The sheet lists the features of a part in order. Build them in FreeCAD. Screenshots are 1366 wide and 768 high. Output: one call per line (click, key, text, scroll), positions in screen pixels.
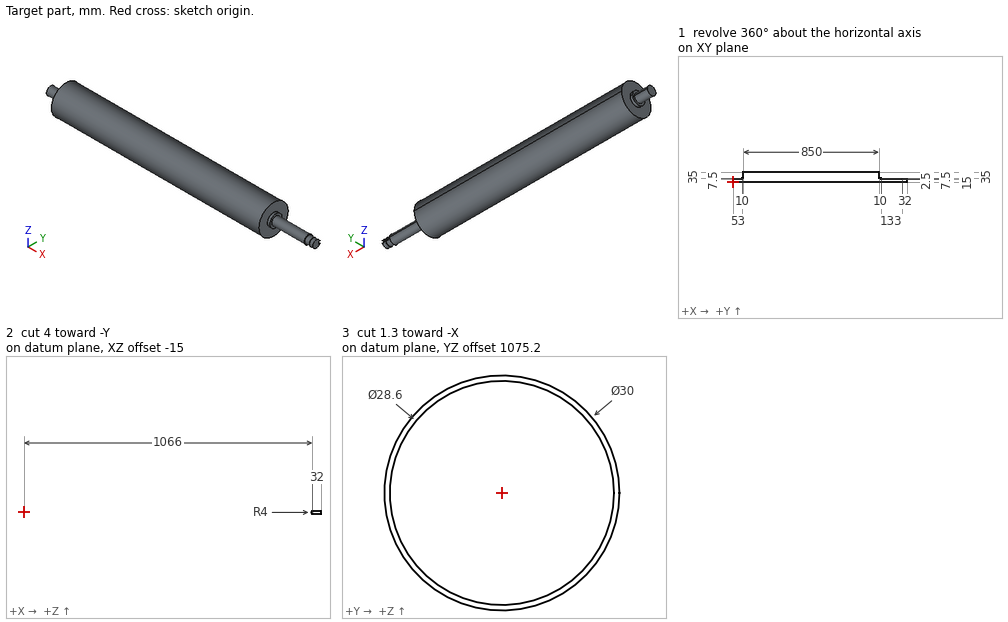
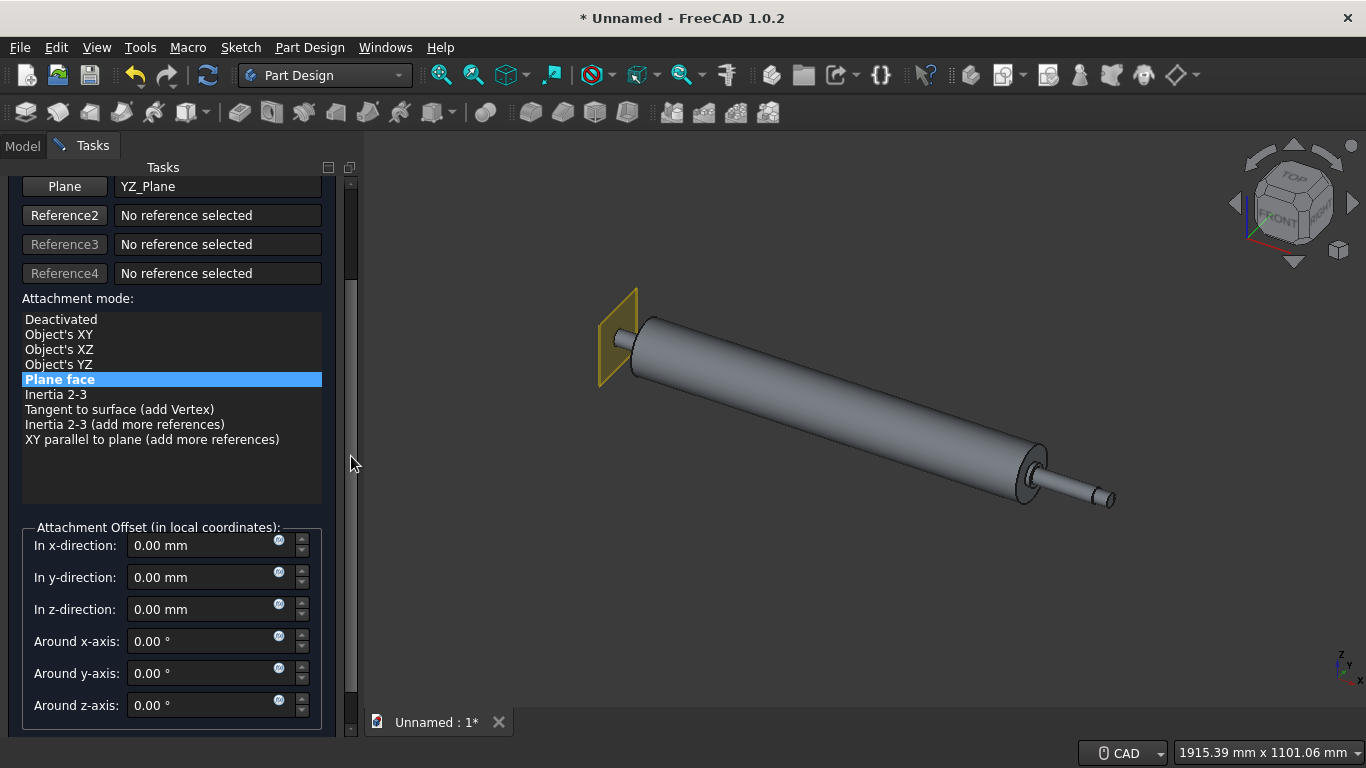
triple_click(210, 609)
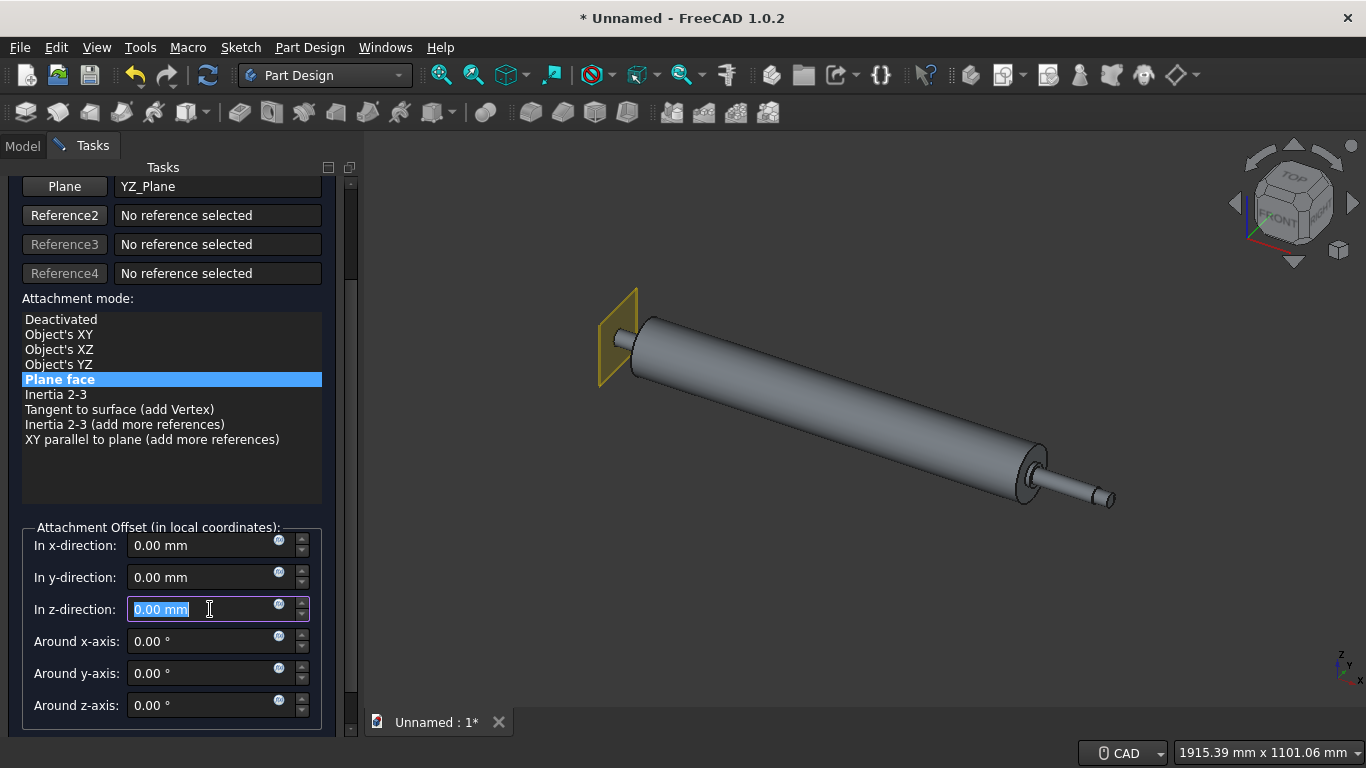
text(1075.2)
key(Tab)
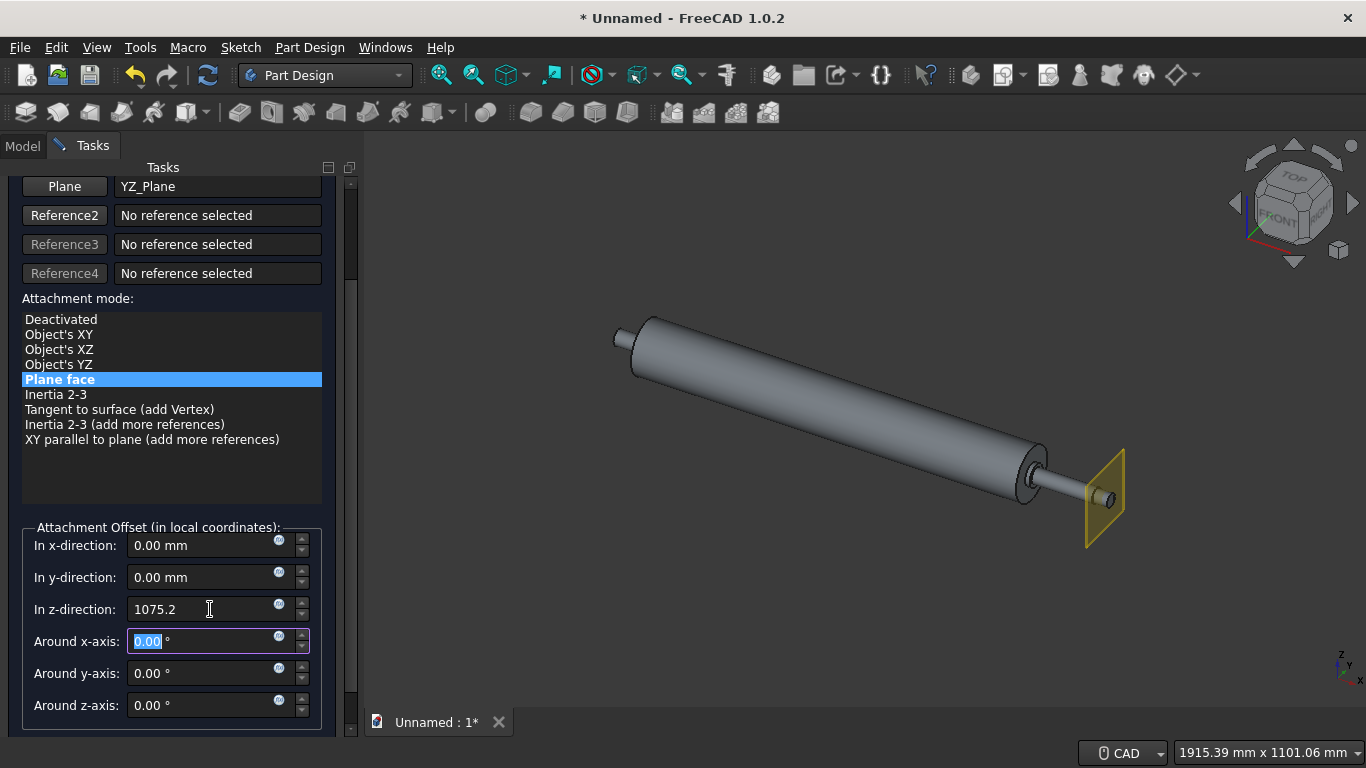
scroll(351, 456, up, 3)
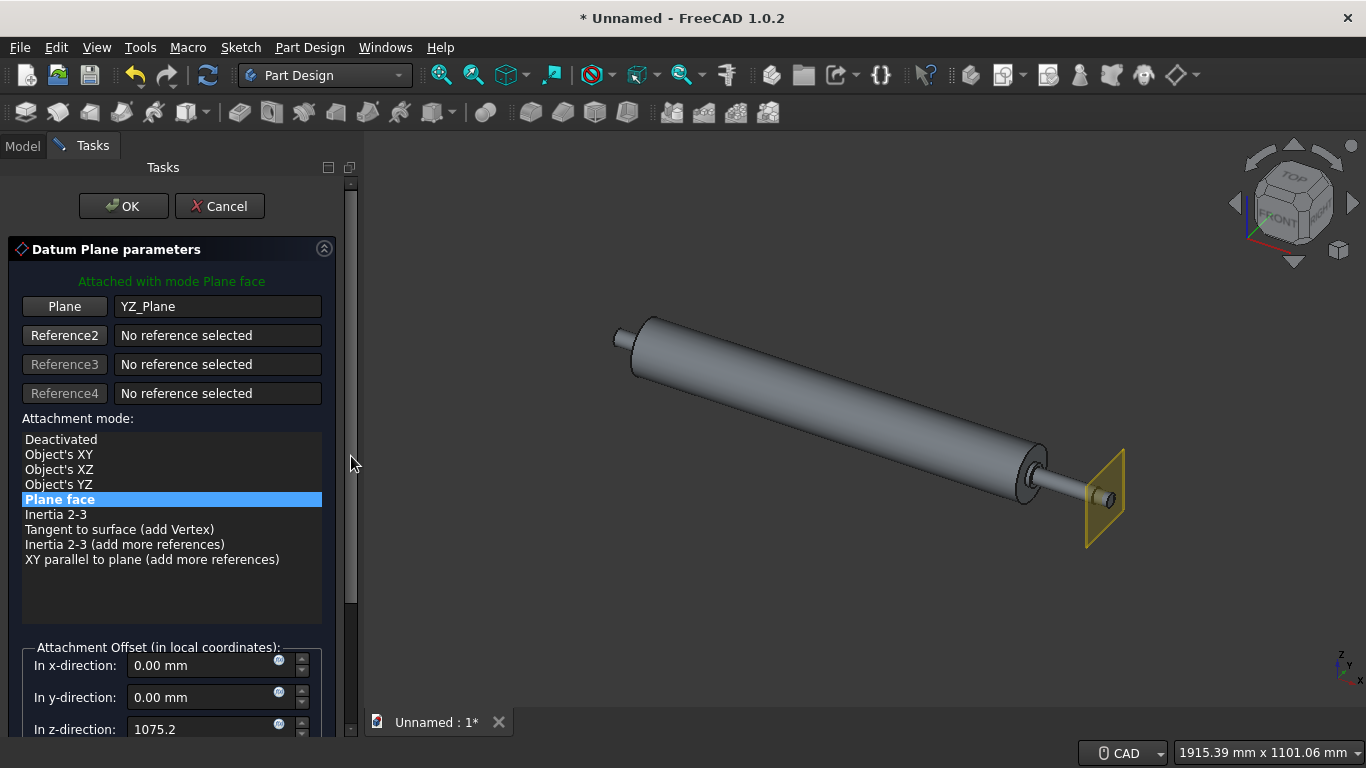
click(124, 206)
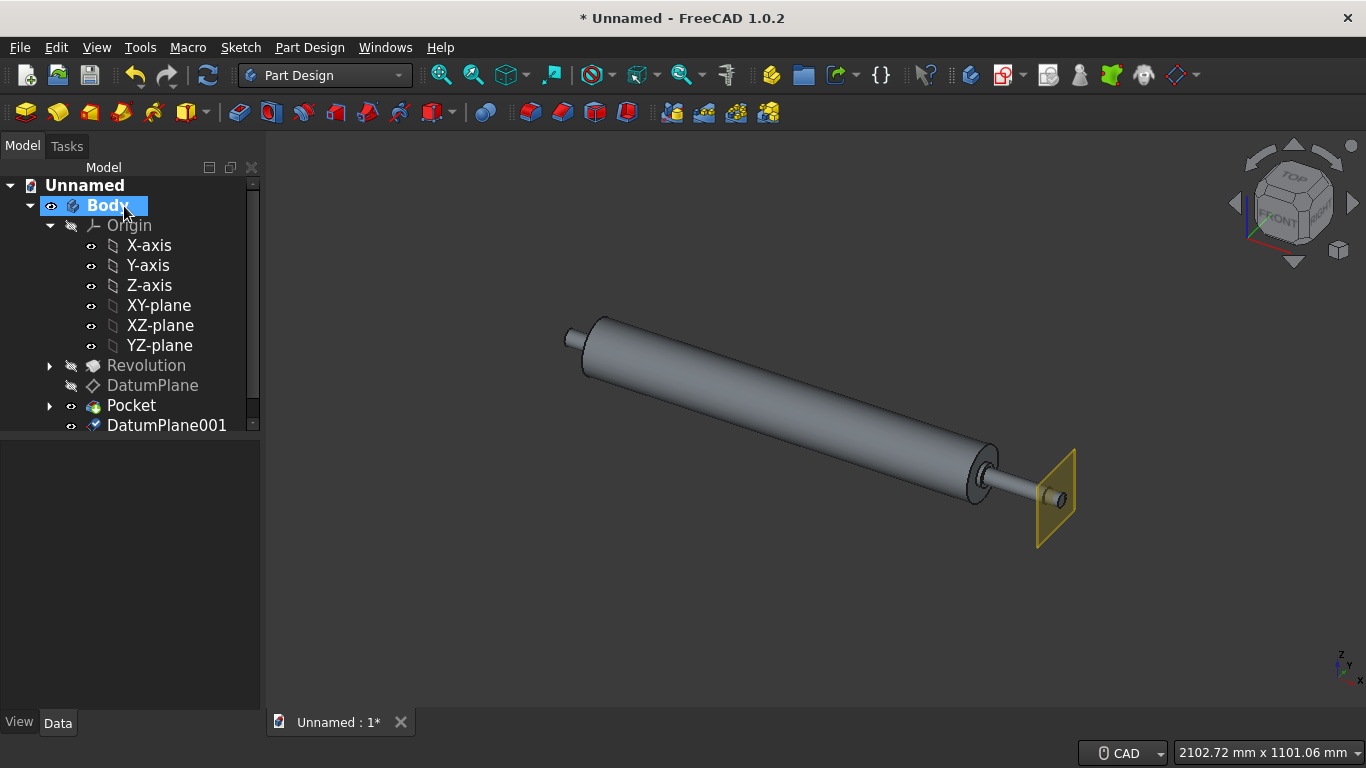
click(116, 426)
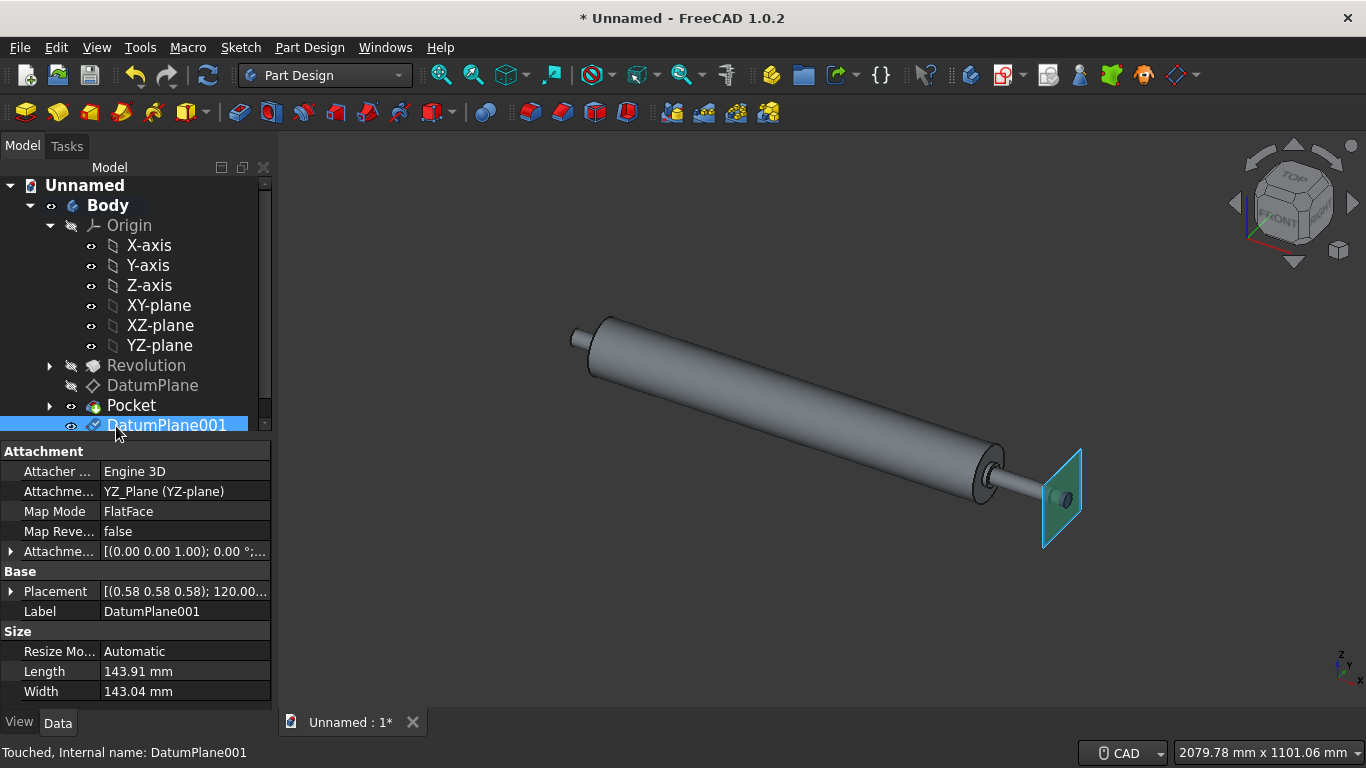
click(1004, 76)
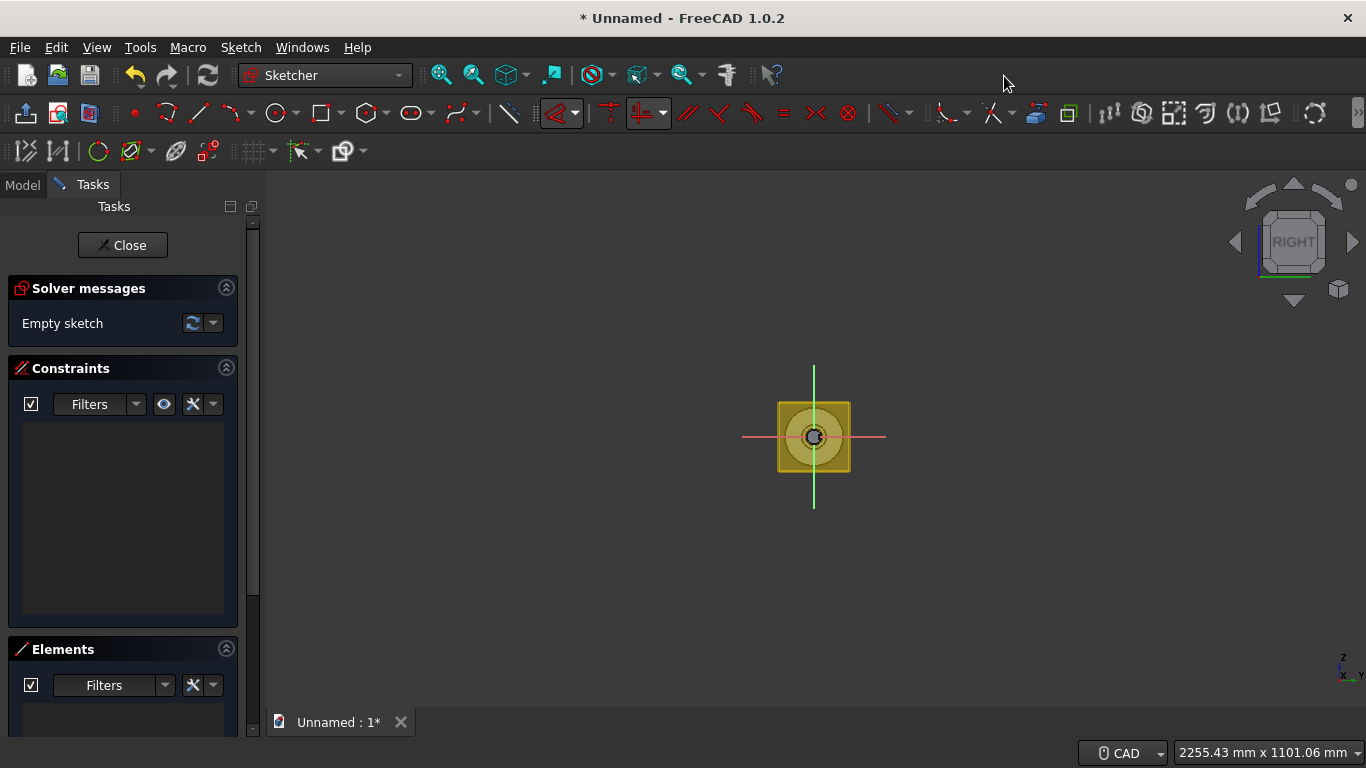
click(90, 114)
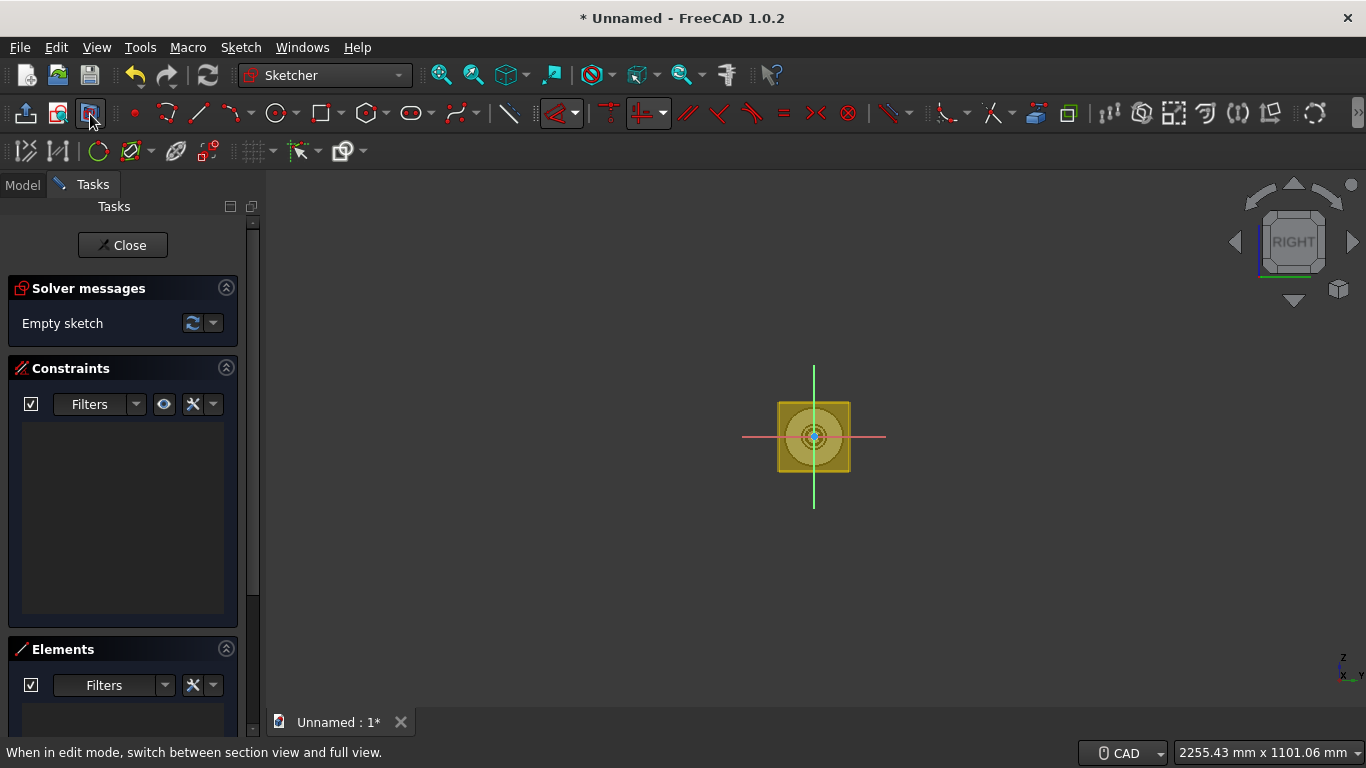
scroll(818, 437, up, 15)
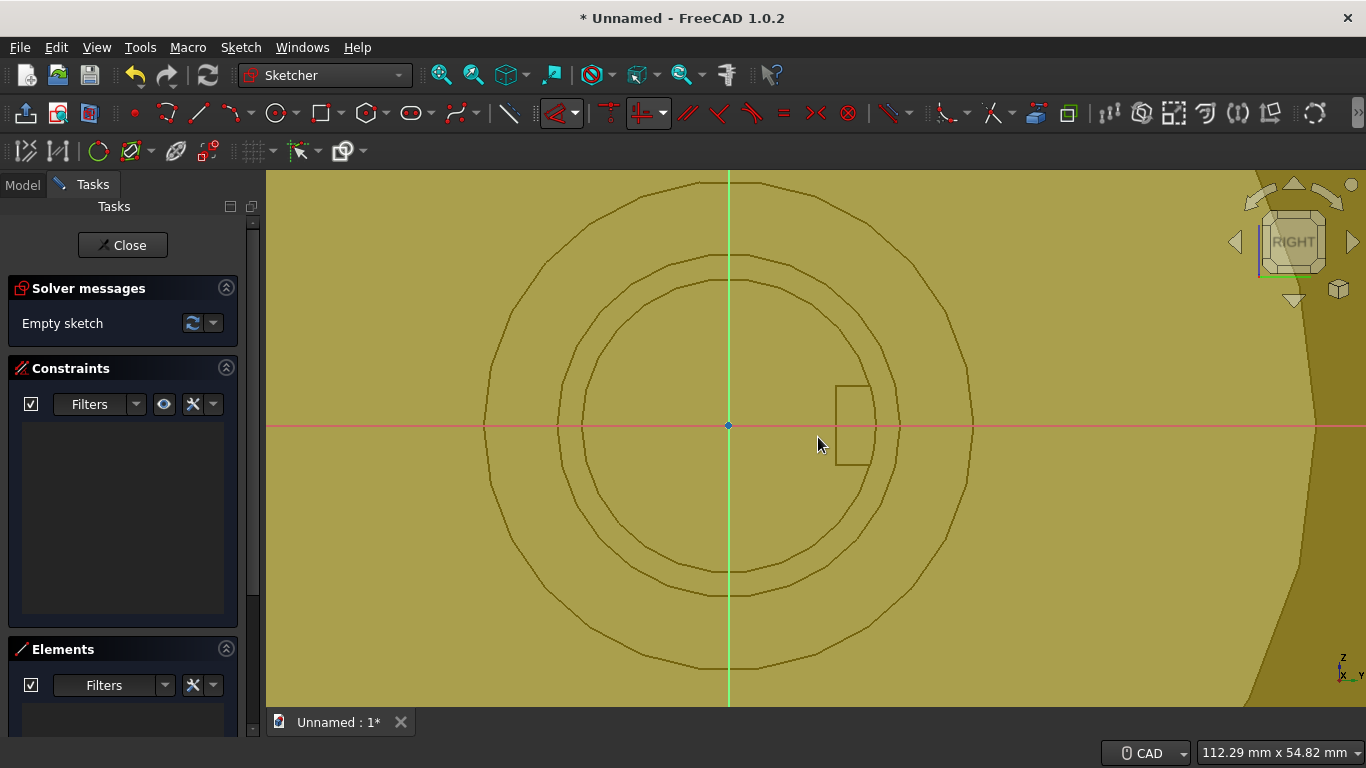
click(276, 114)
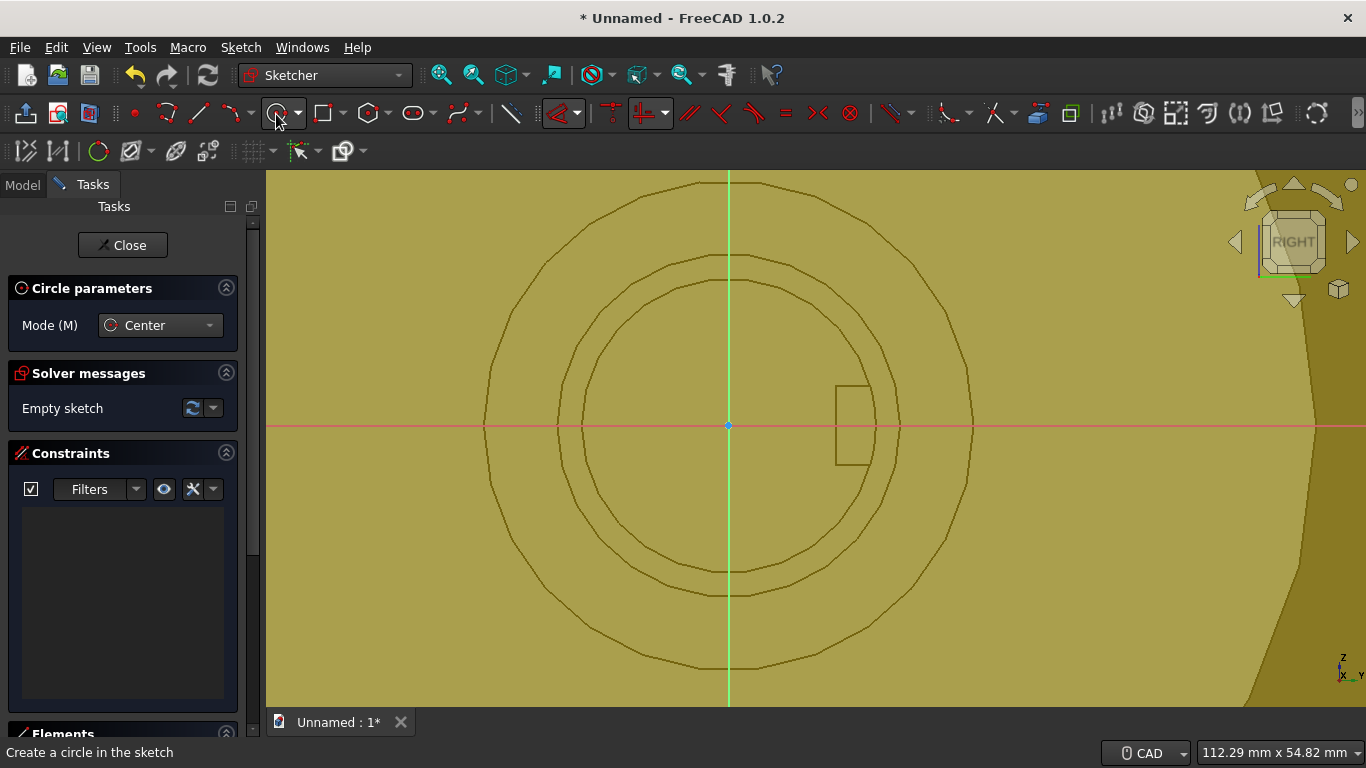
click(729, 426)
move(833, 322)